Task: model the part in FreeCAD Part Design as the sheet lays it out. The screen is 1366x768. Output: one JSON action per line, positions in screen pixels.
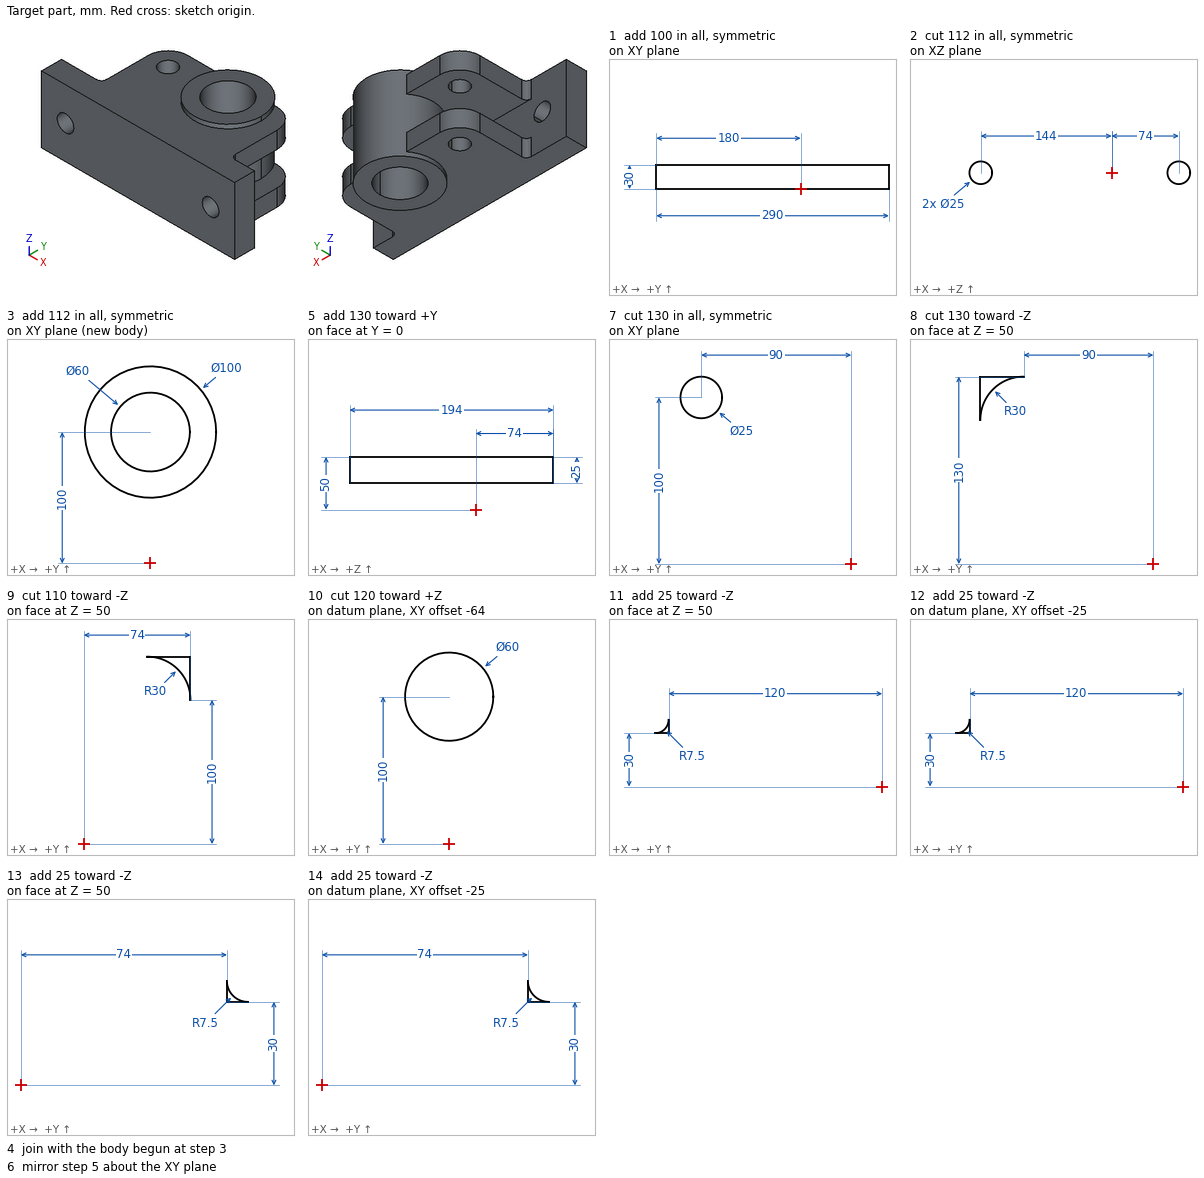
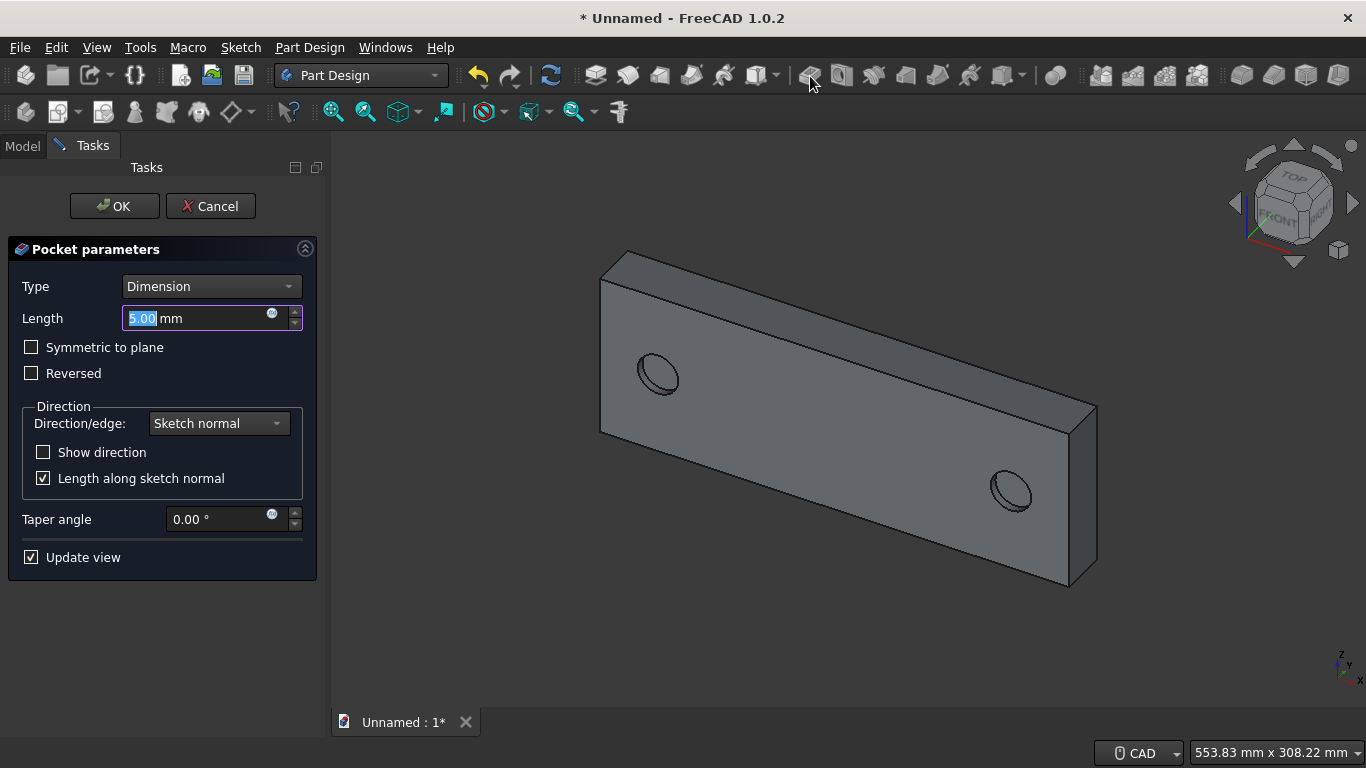
{"action": "type", "text": "112"}
{"action": "key", "text": "Tab"}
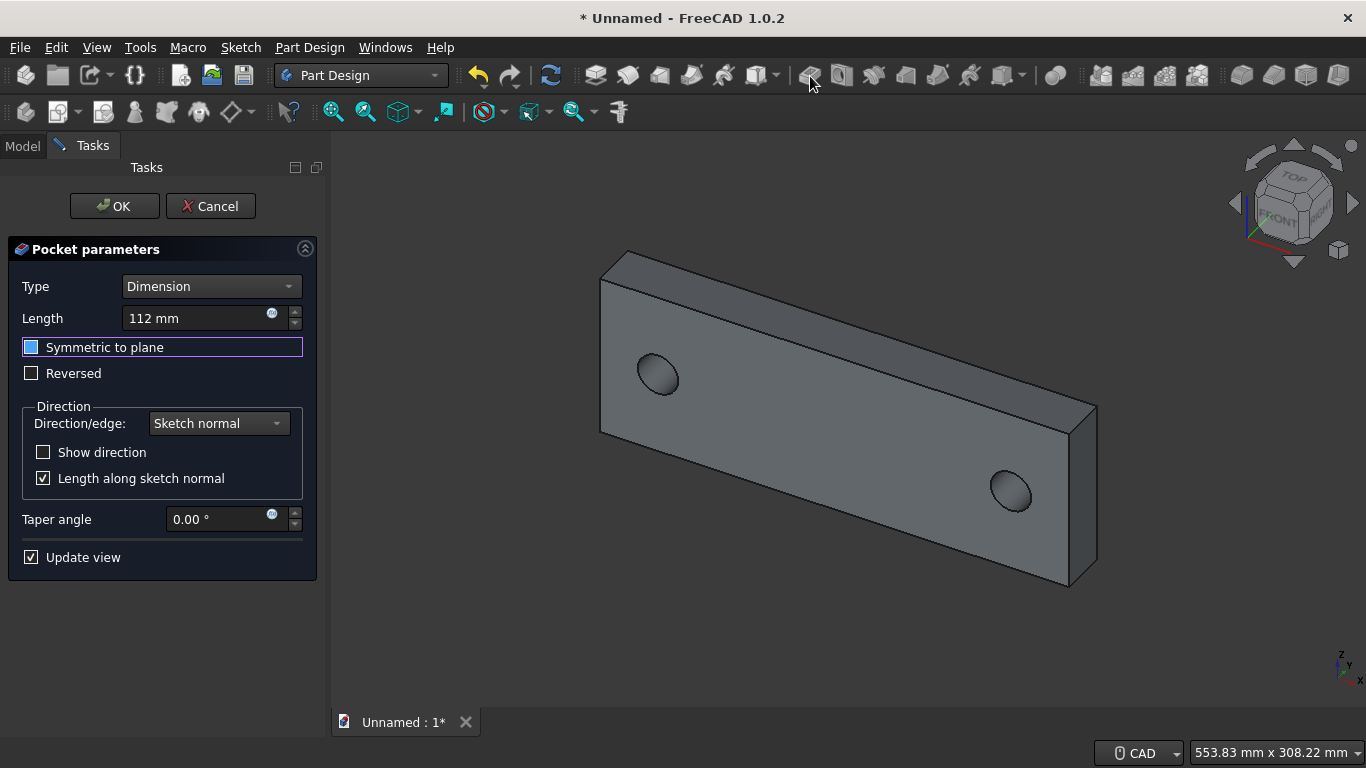
{"action": "left_click", "coordinate": [30, 347]}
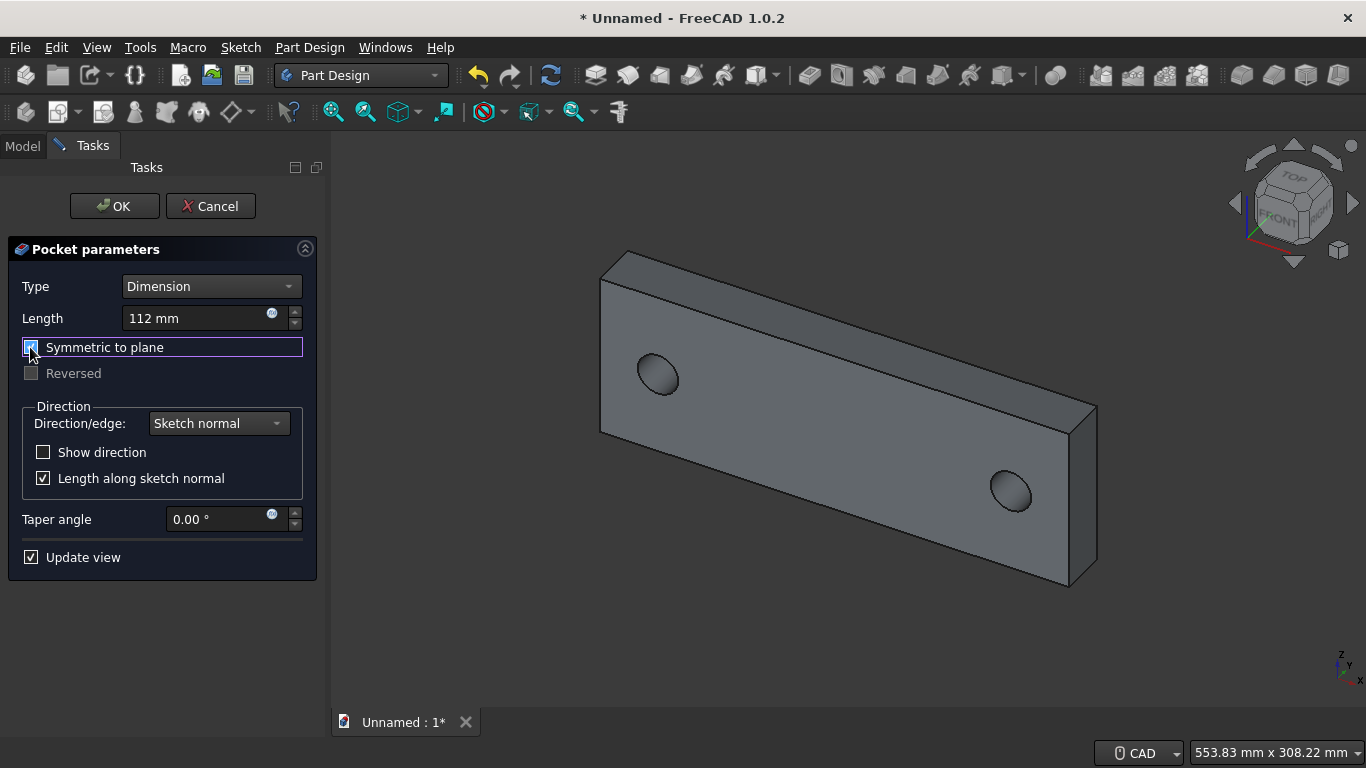
{"action": "left_click", "coordinate": [115, 206]}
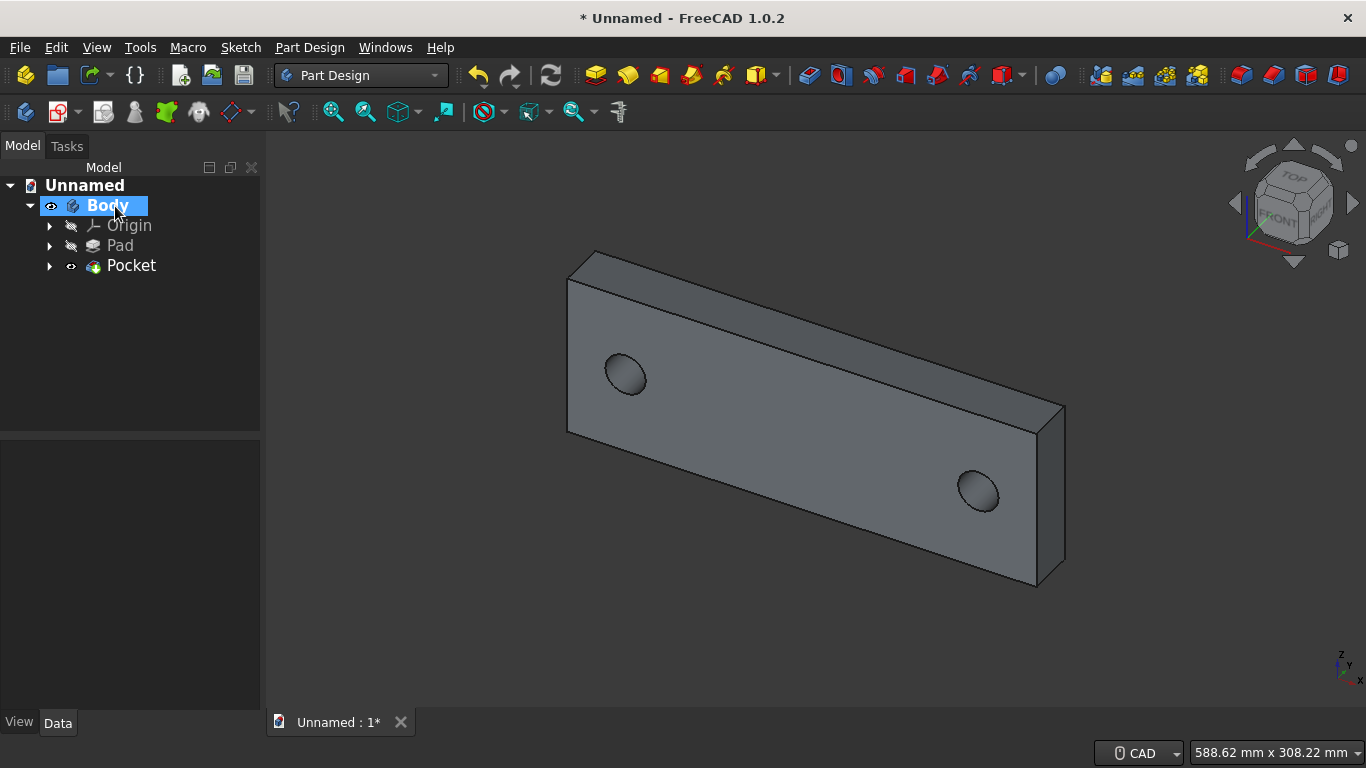
{"action": "left_click", "coordinate": [26, 112]}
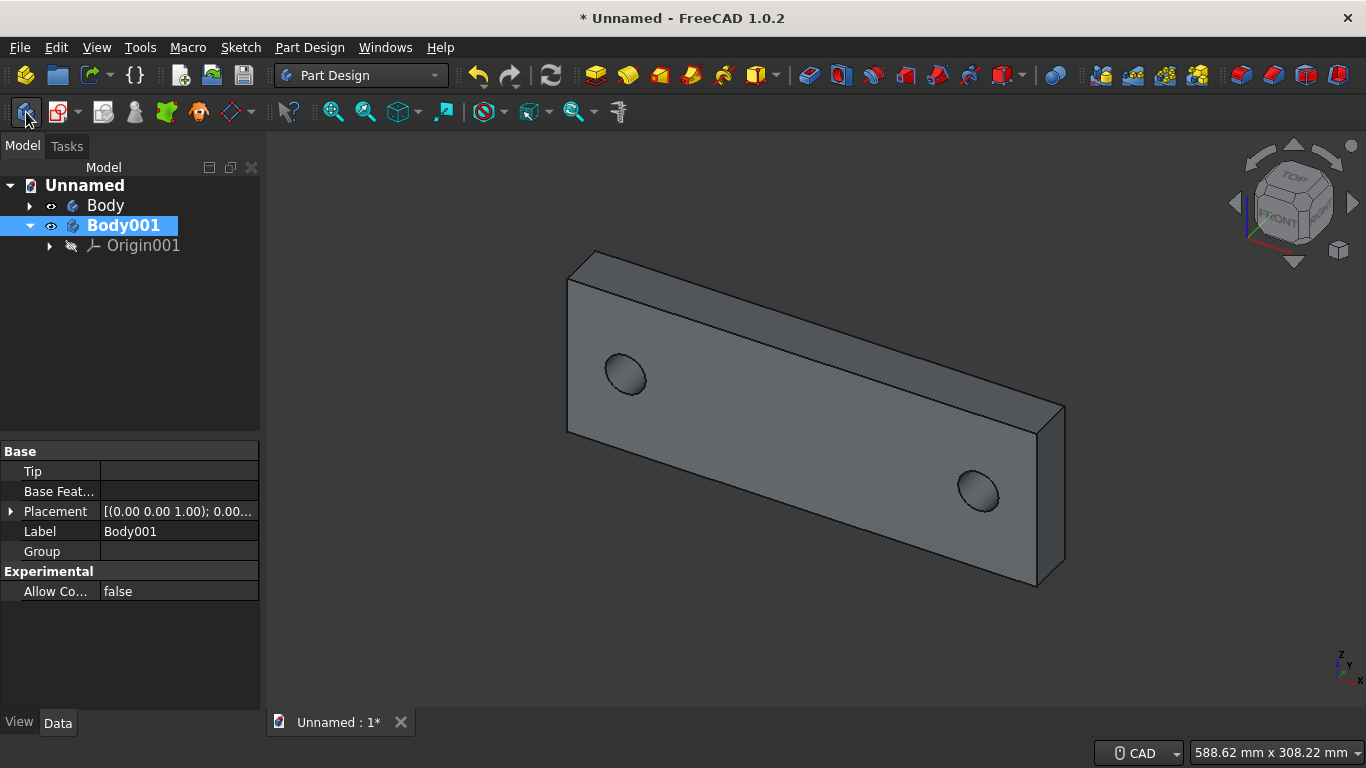
{"action": "left_click", "coordinate": [306, 667]}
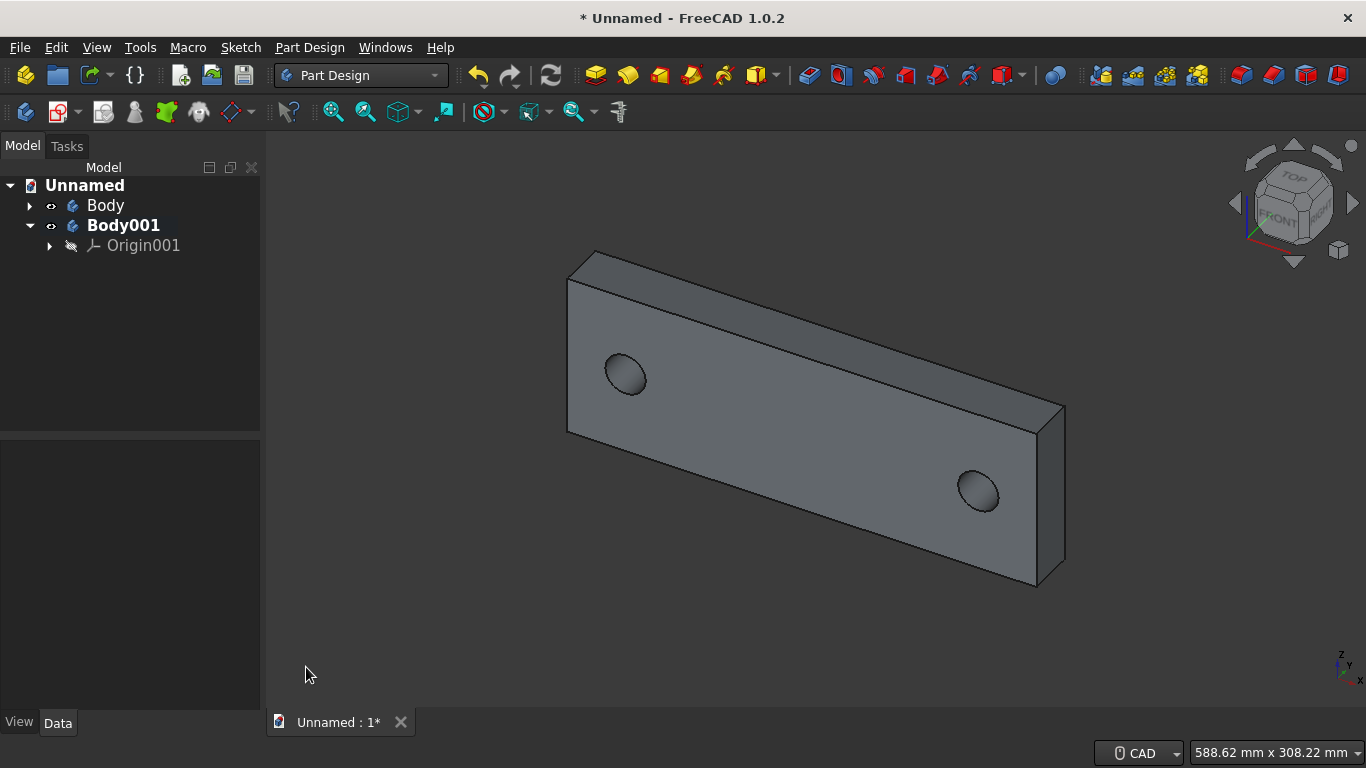
{"action": "left_click", "coordinate": [58, 112]}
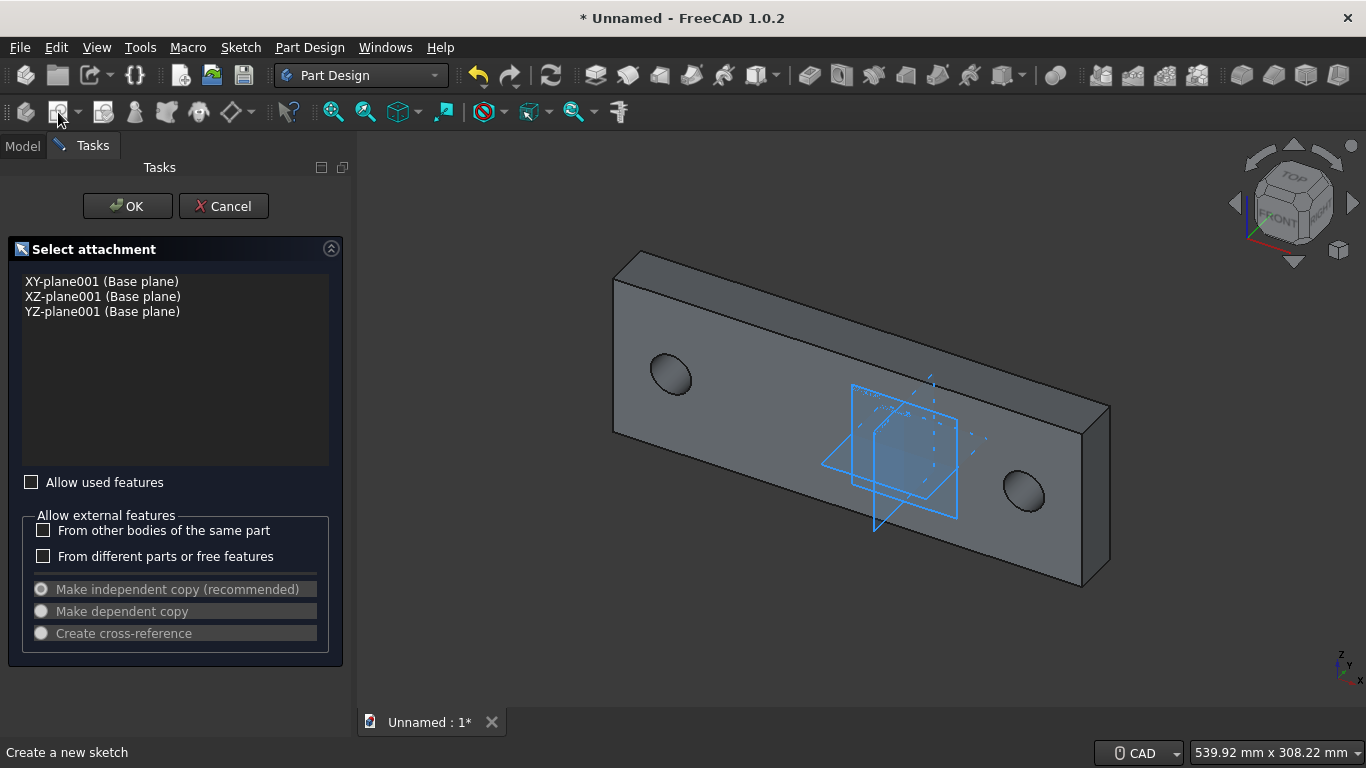
{"action": "left_click", "coordinate": [82, 282]}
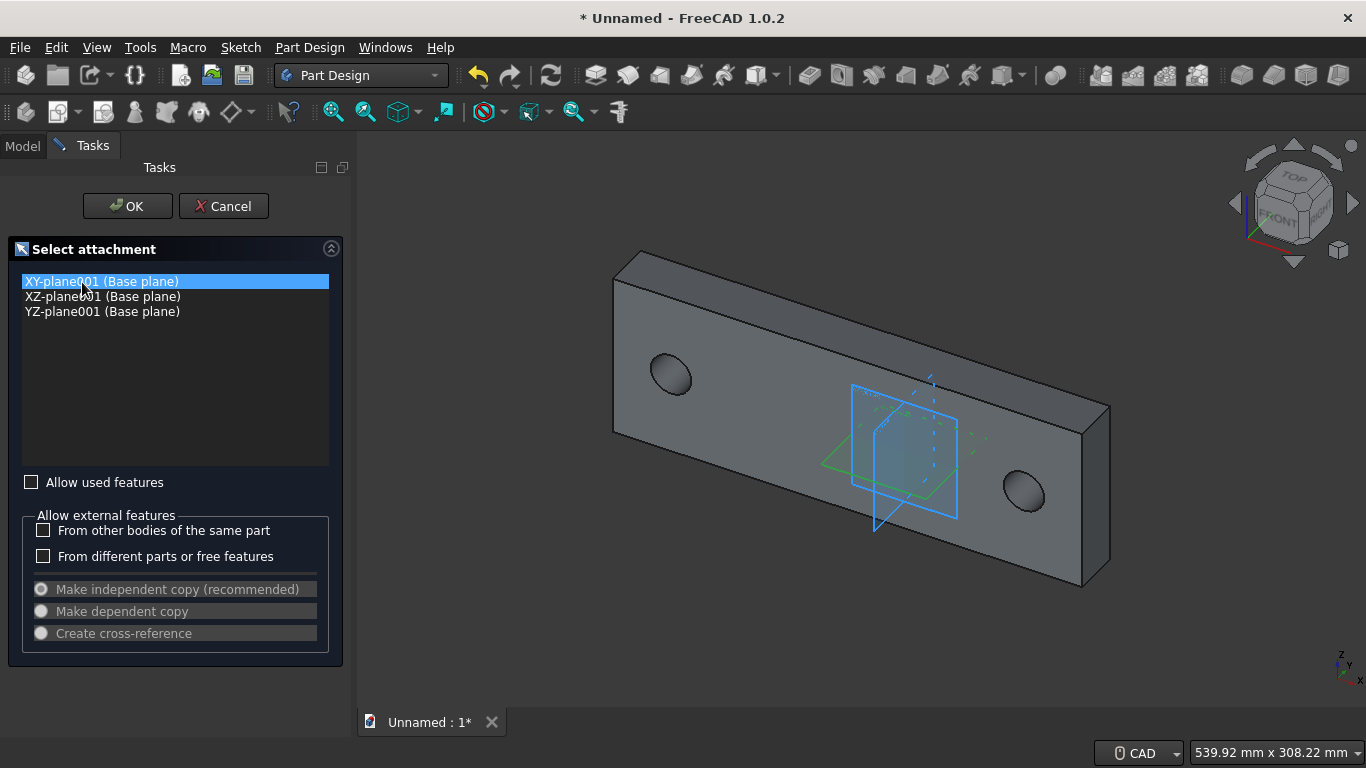
{"action": "left_click", "coordinate": [128, 206]}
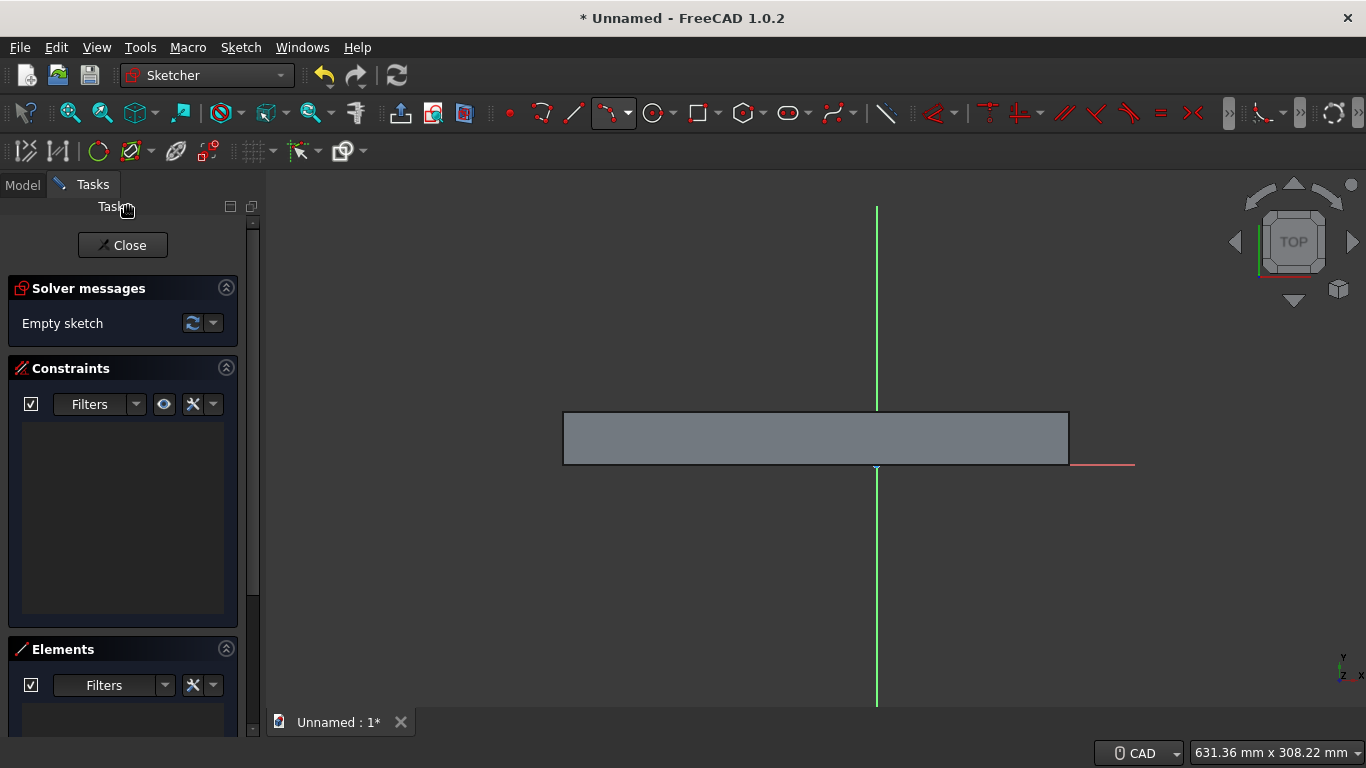
{"action": "scroll", "coordinate": [294, 679], "scroll_direction": "down", "scroll_amount": 1}